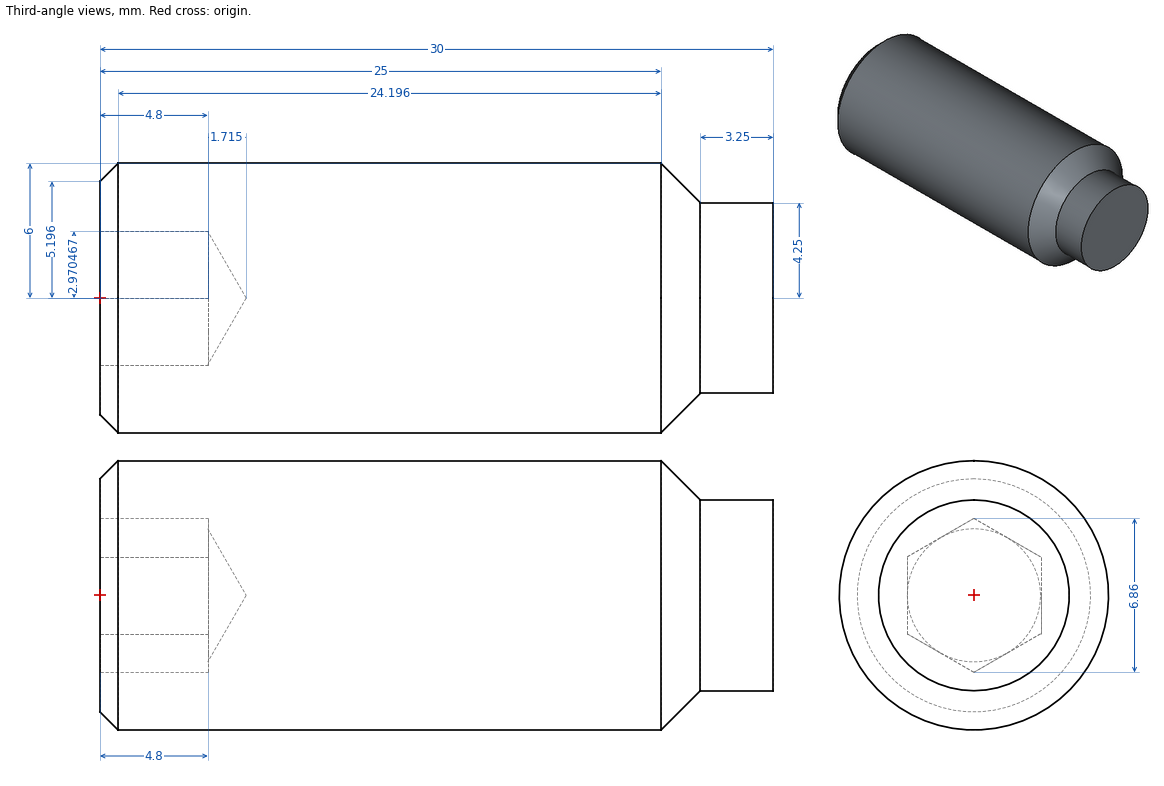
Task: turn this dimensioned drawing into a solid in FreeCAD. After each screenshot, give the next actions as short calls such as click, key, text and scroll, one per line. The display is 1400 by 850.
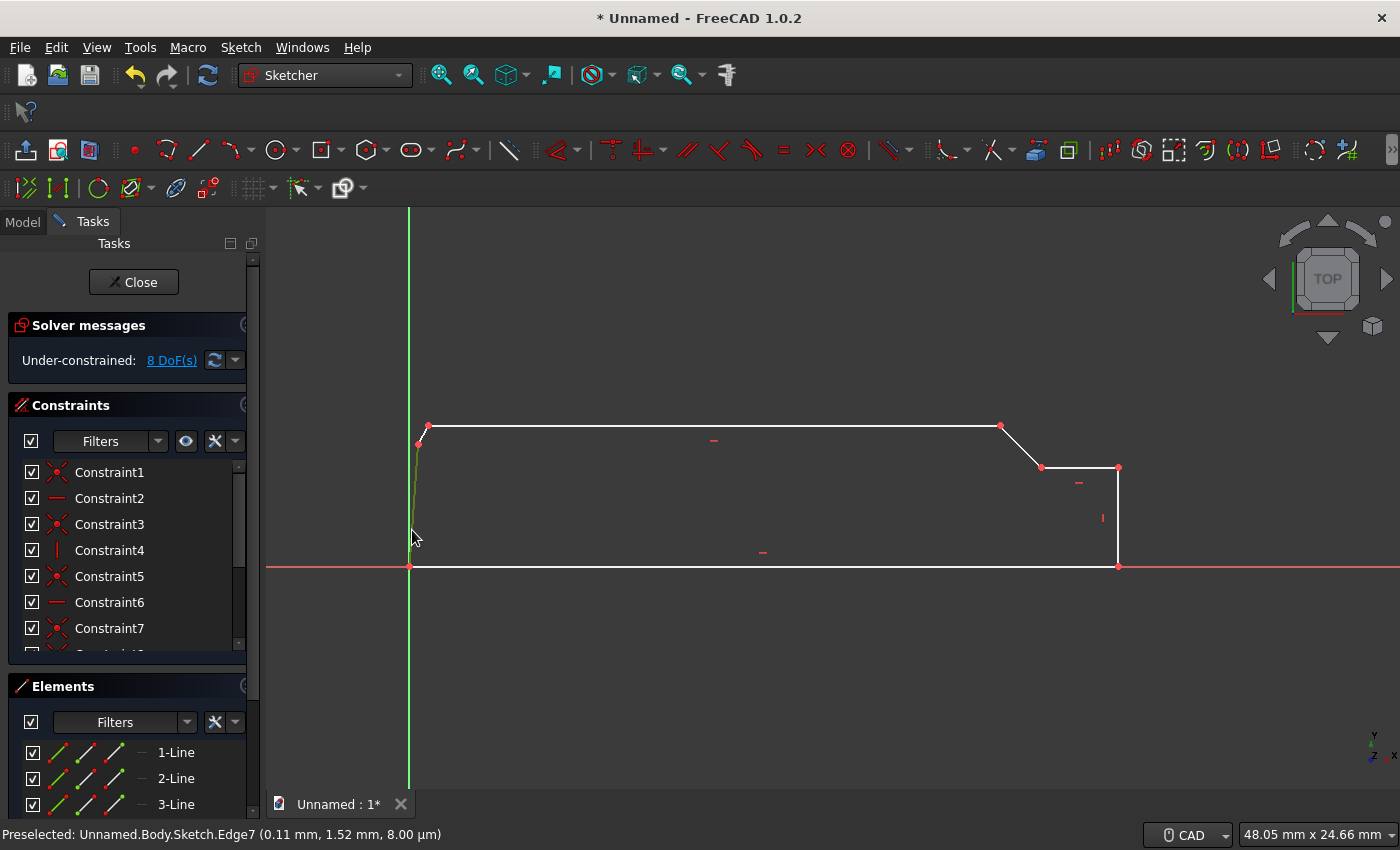
click(666, 150)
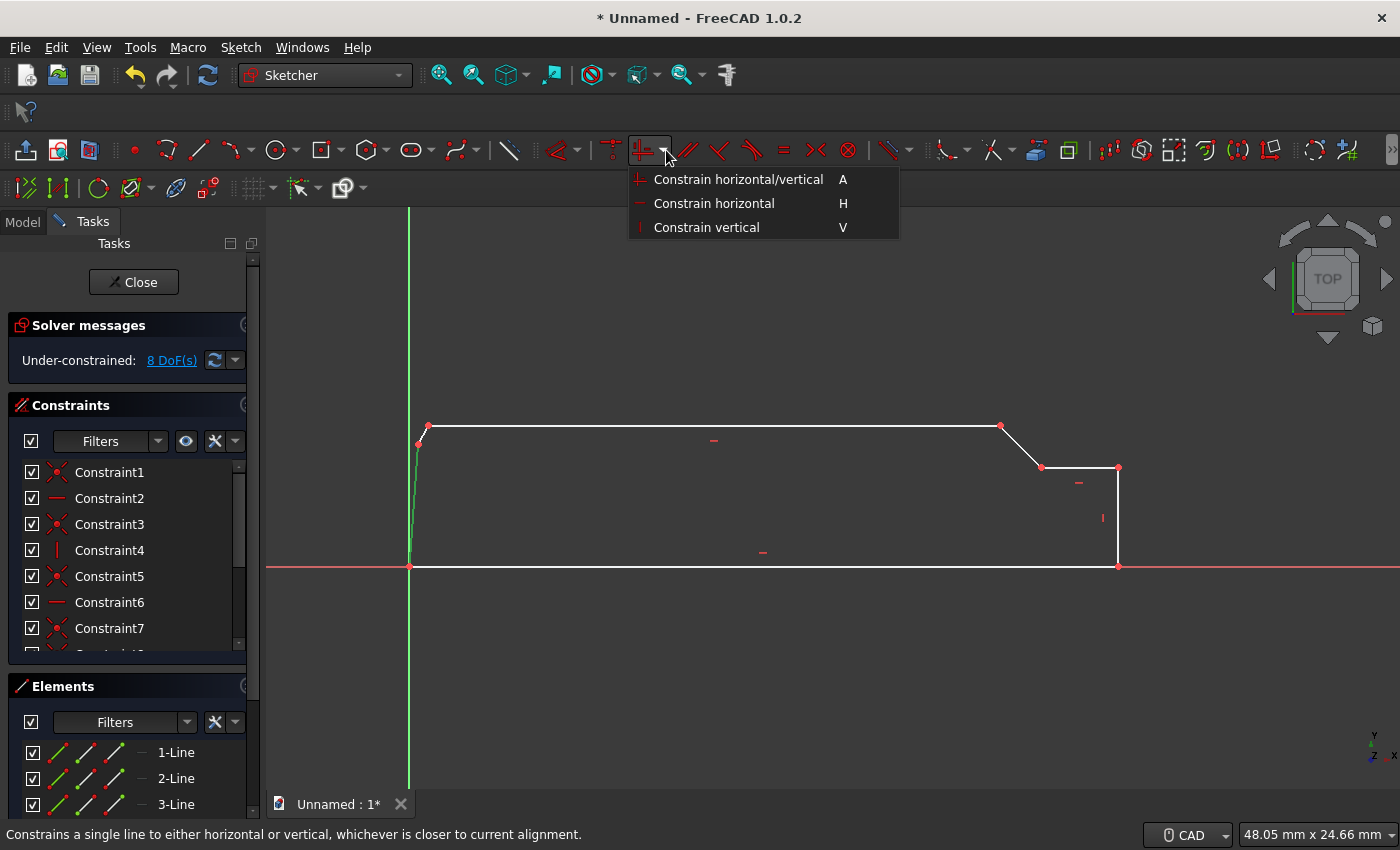
click(764, 227)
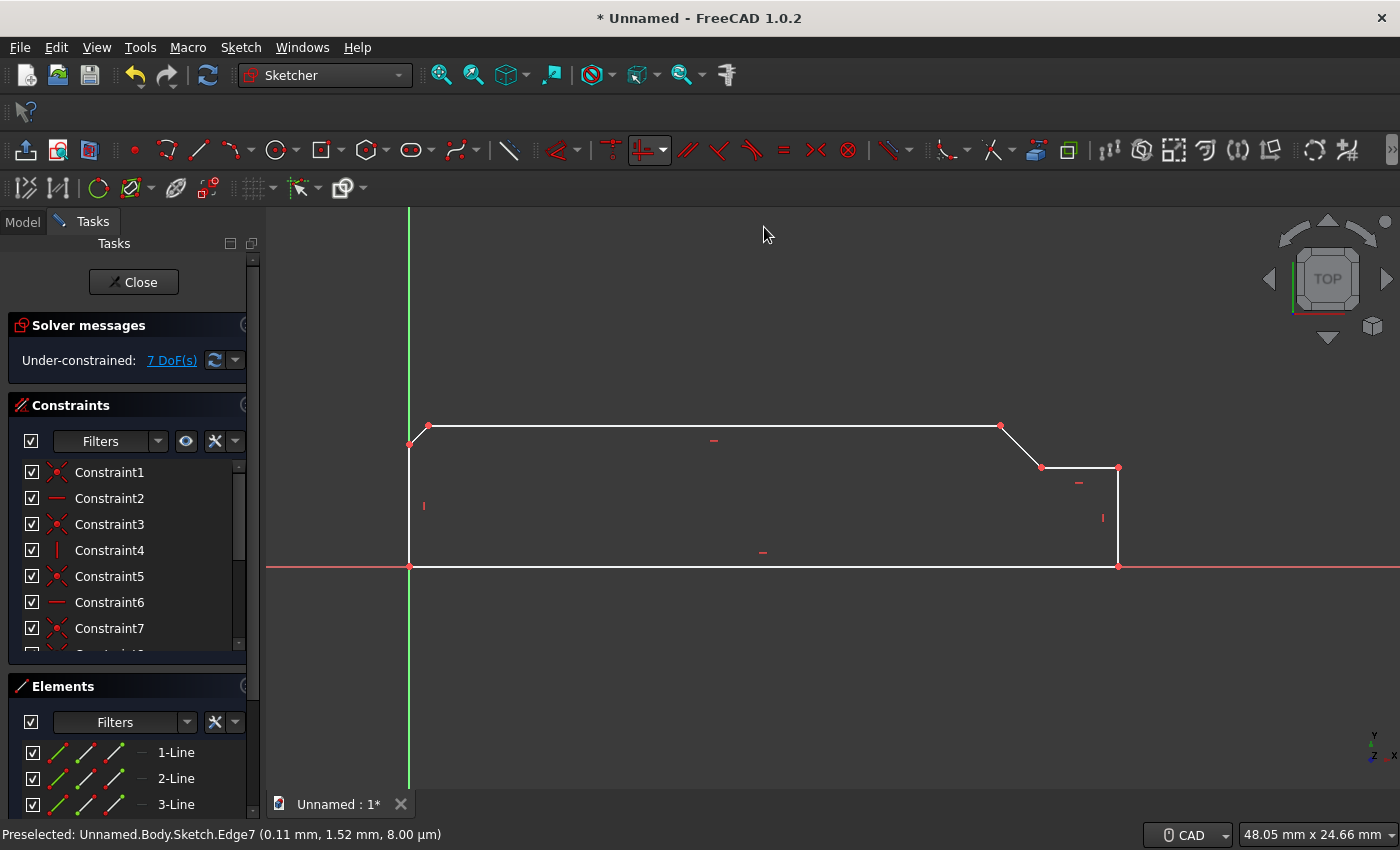
click(556, 150)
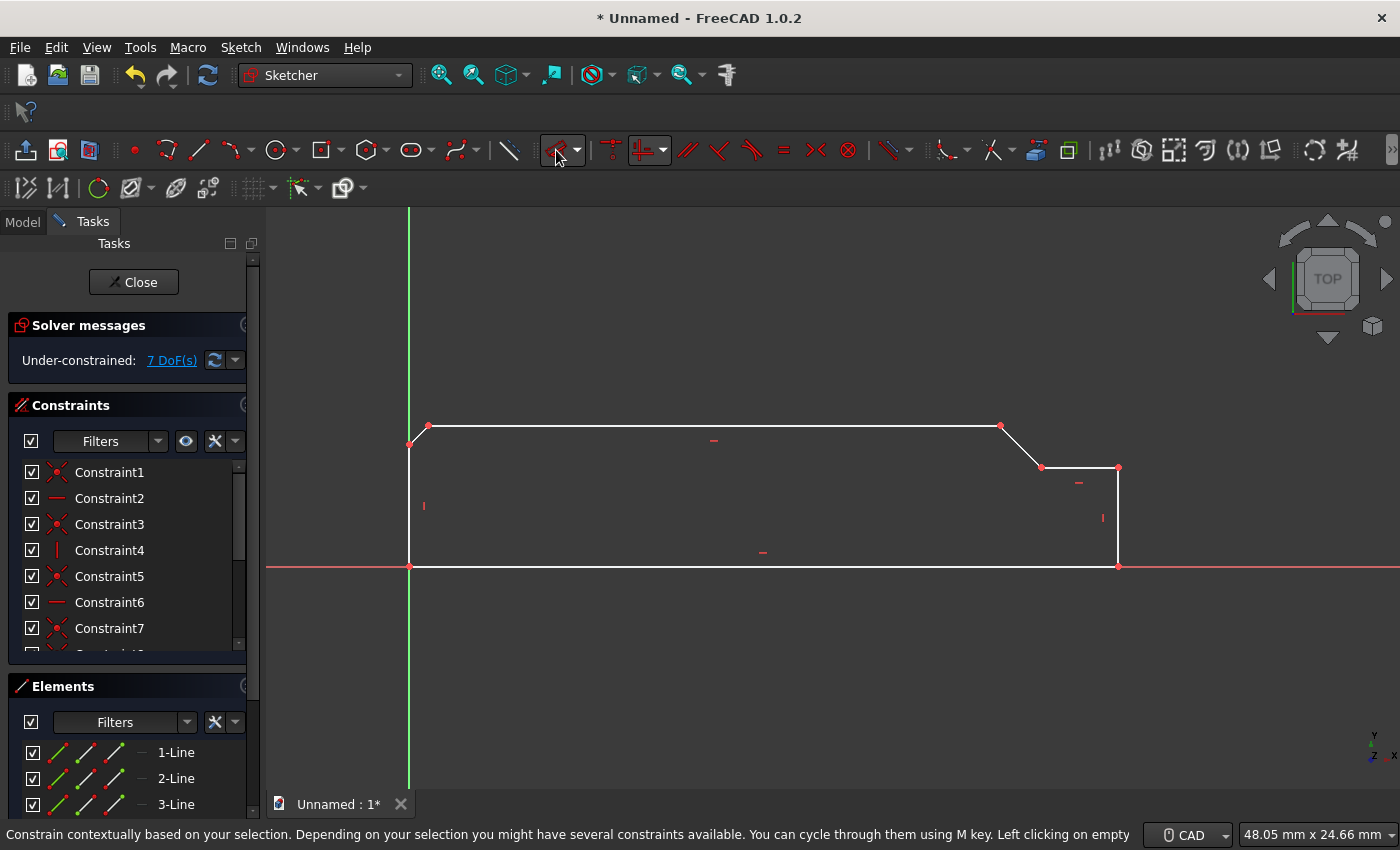
click(622, 567)
click(764, 601)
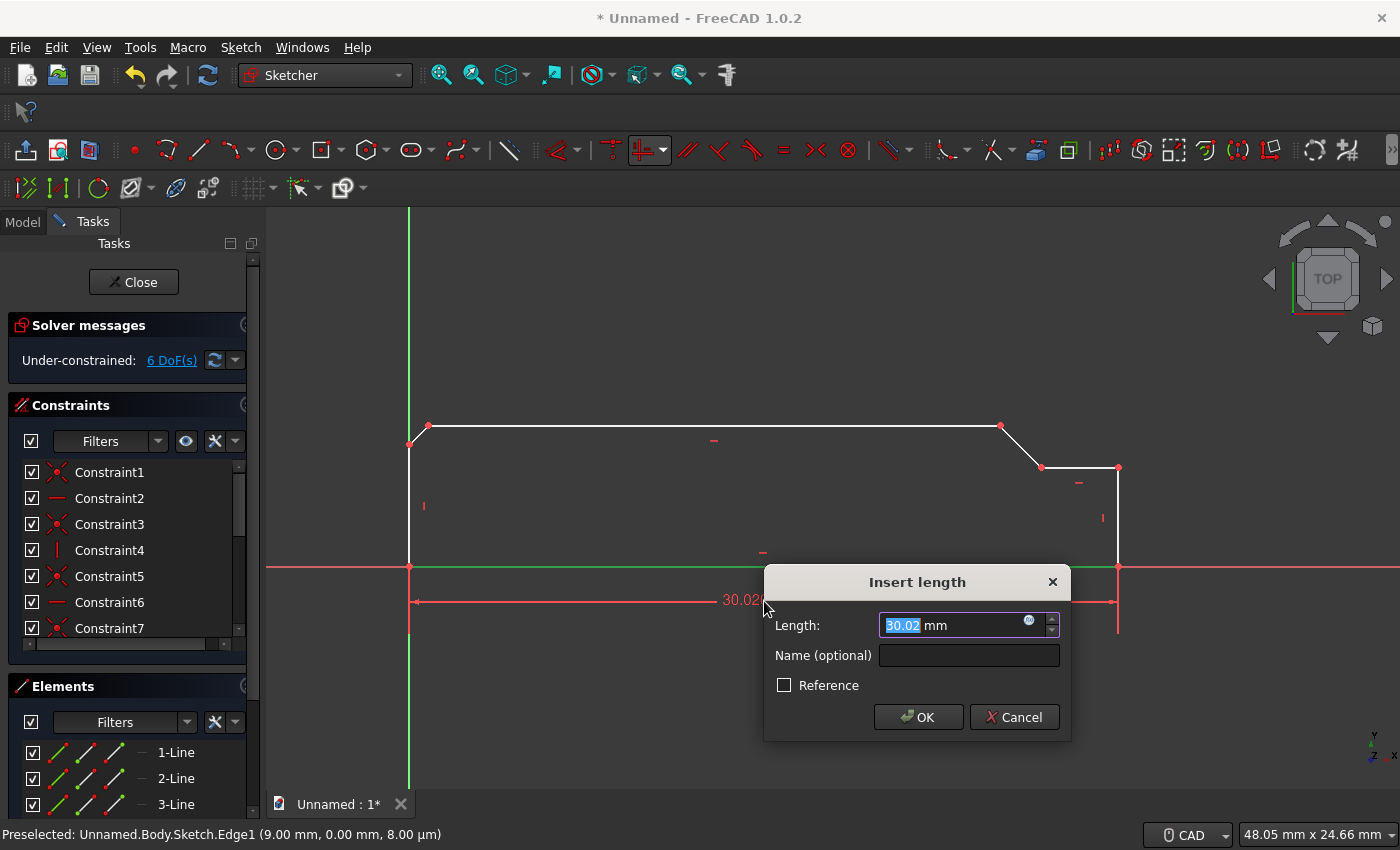
text(30)
key(Return)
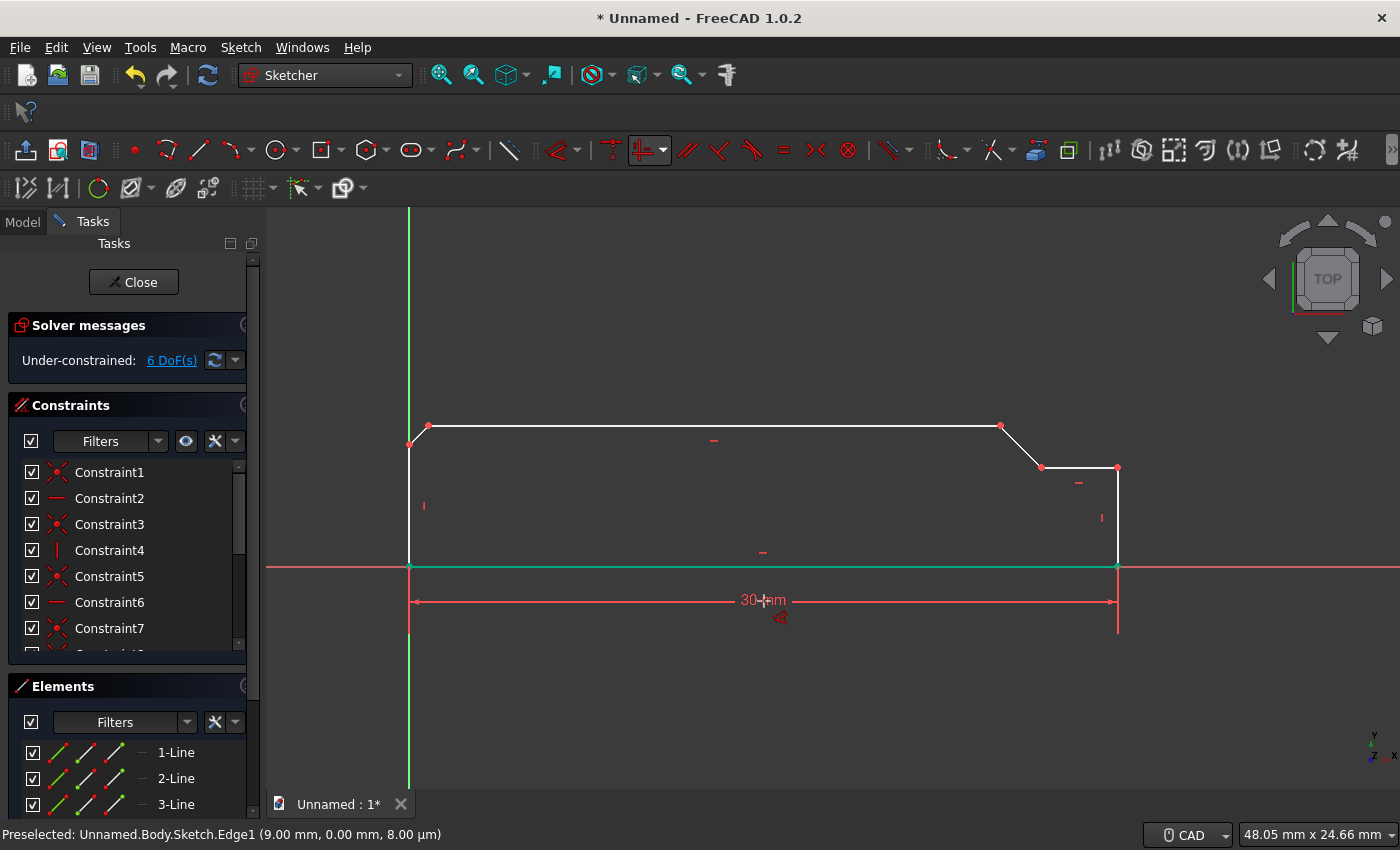
click(1000, 426)
click(375, 496)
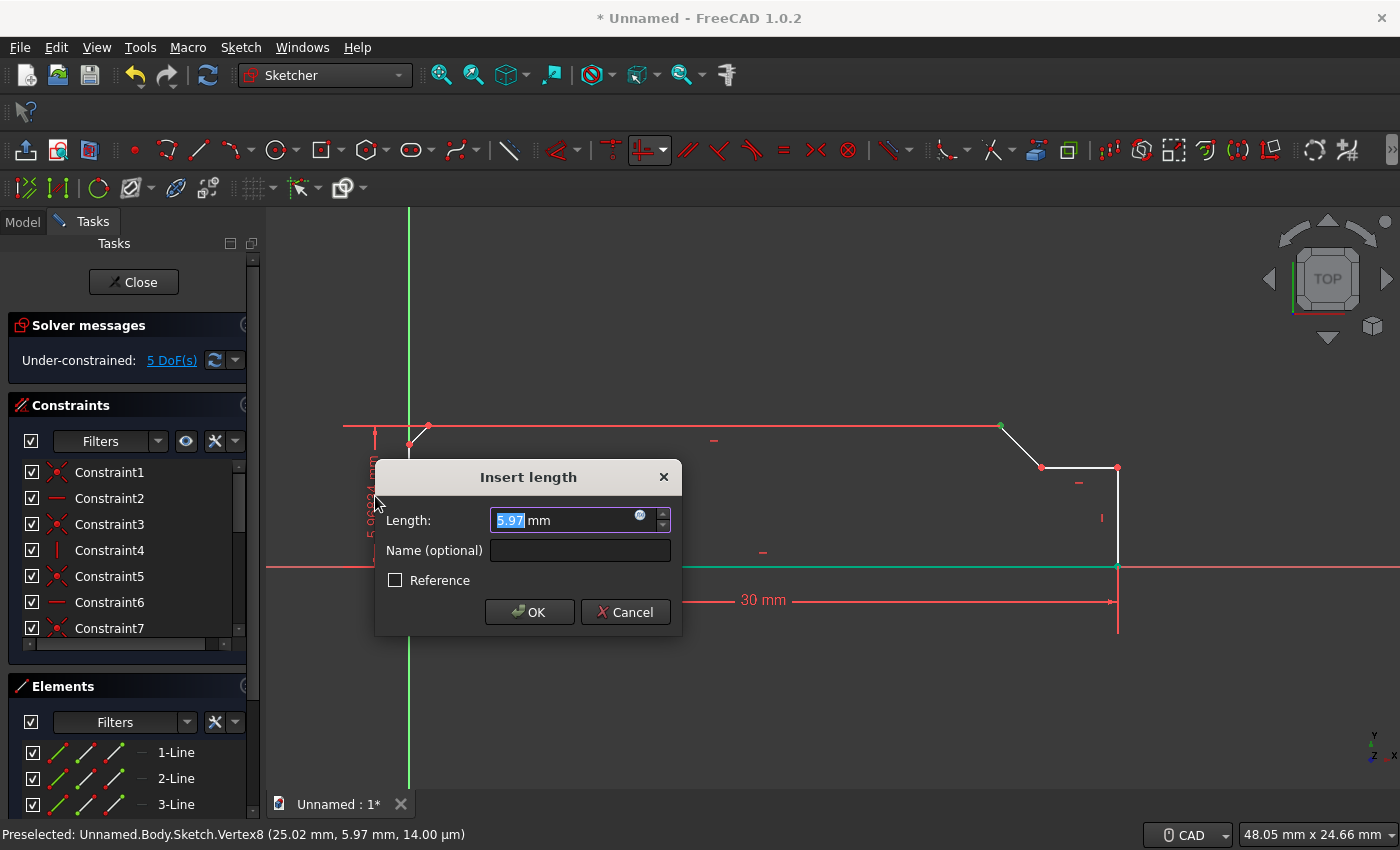
text(6)
key(Return)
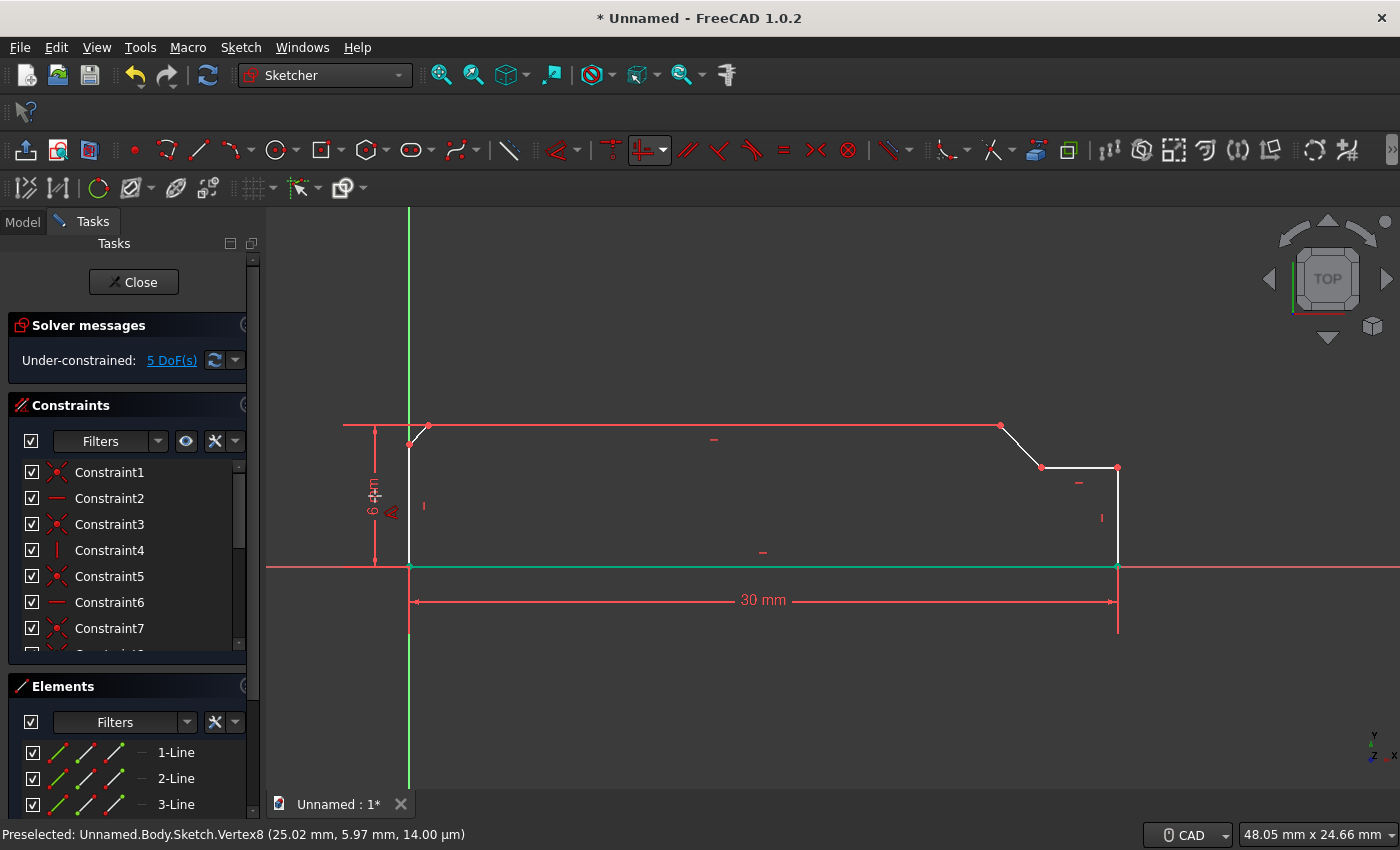
click(1000, 425)
click(569, 601)